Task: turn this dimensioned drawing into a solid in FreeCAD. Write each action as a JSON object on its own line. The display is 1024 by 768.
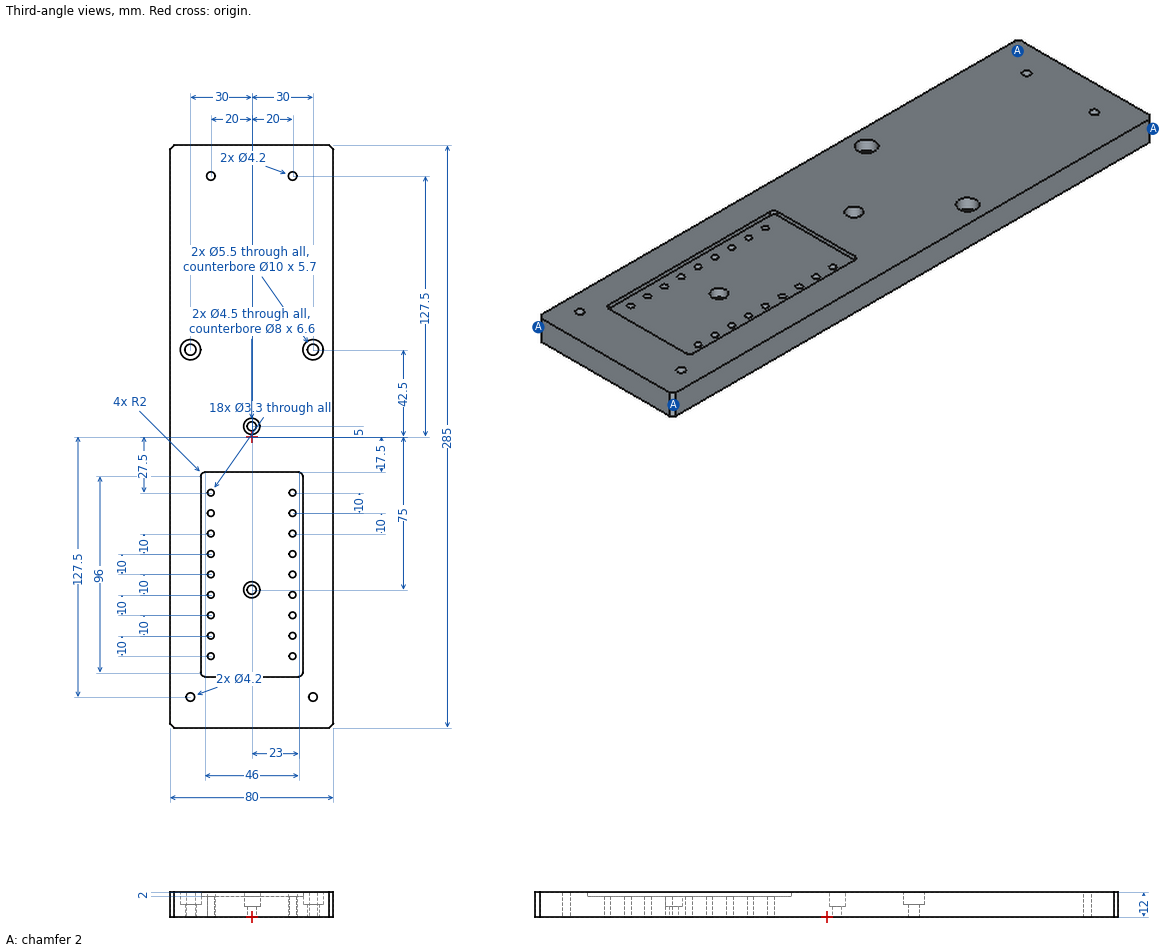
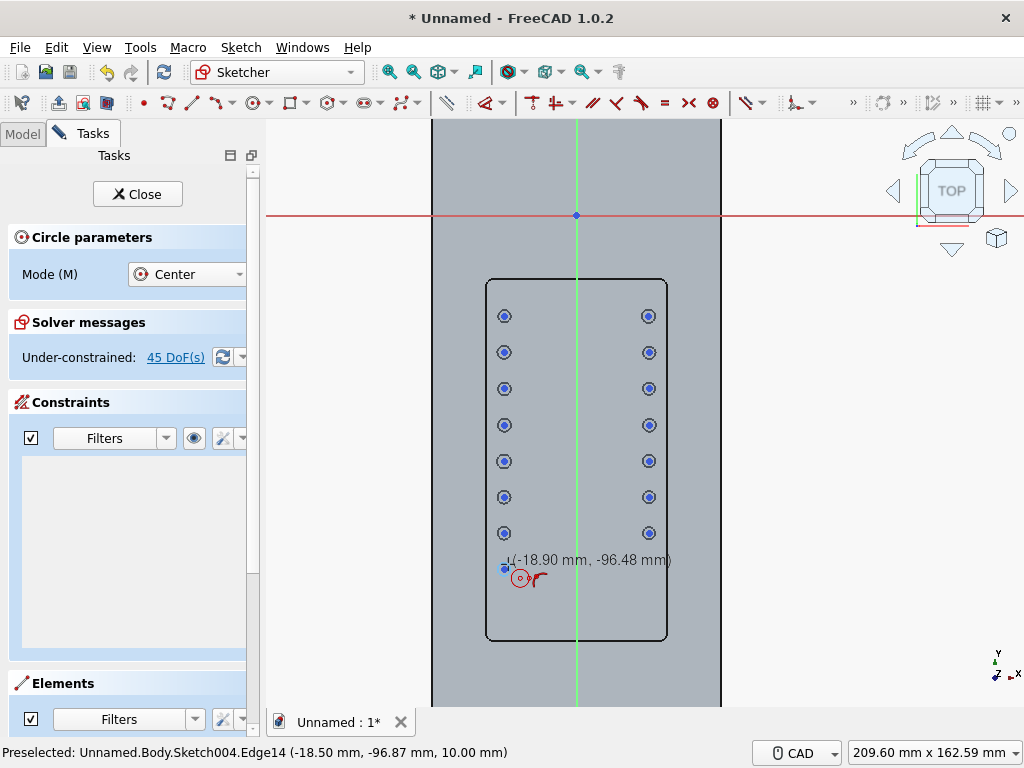
{"action": "scroll", "coordinate": [649, 569], "scroll_direction": "up", "scroll_amount": 7}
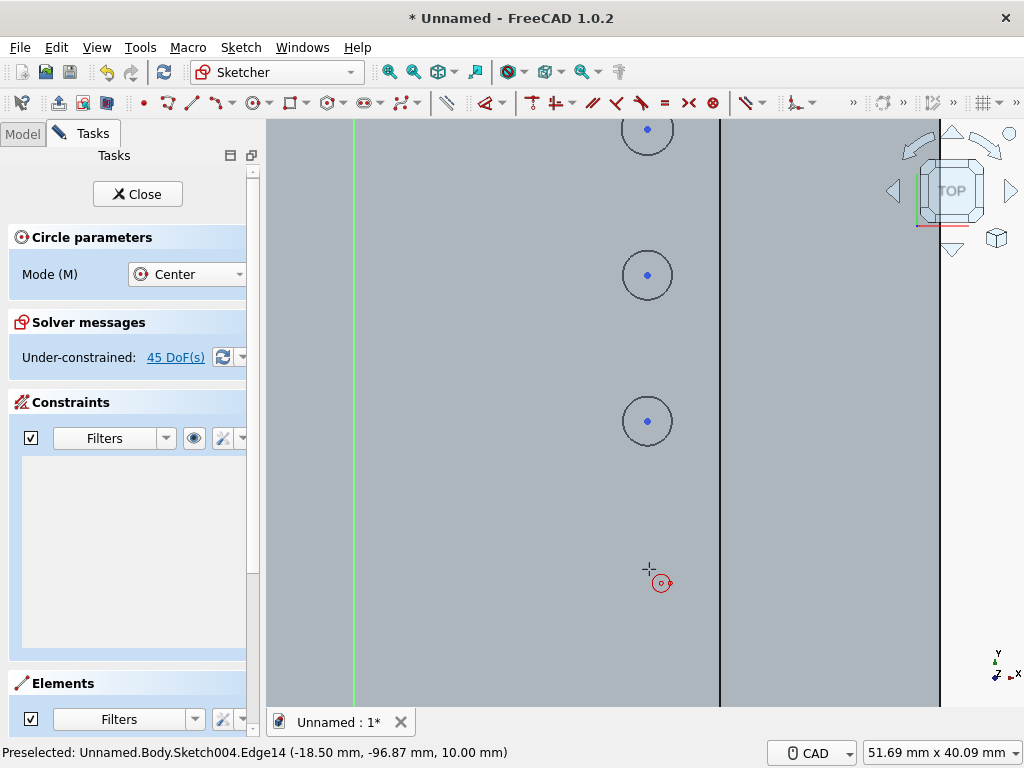
{"action": "scroll", "coordinate": [649, 569], "scroll_direction": "down", "scroll_amount": 7}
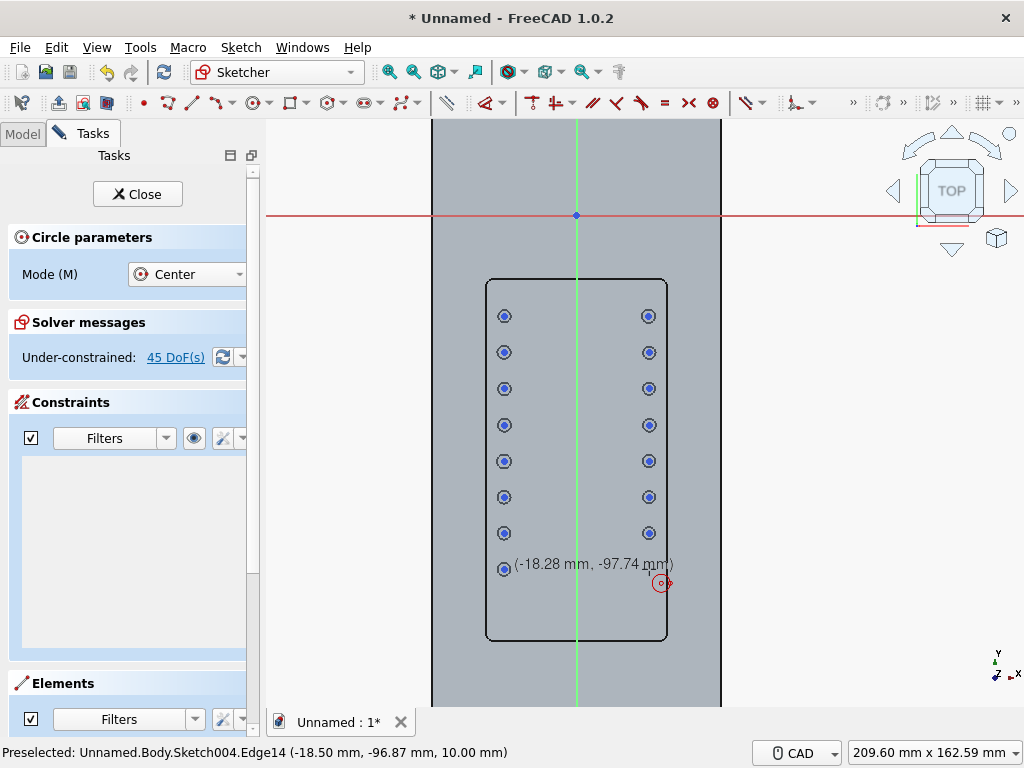
{"action": "left_click", "coordinate": [649, 569]}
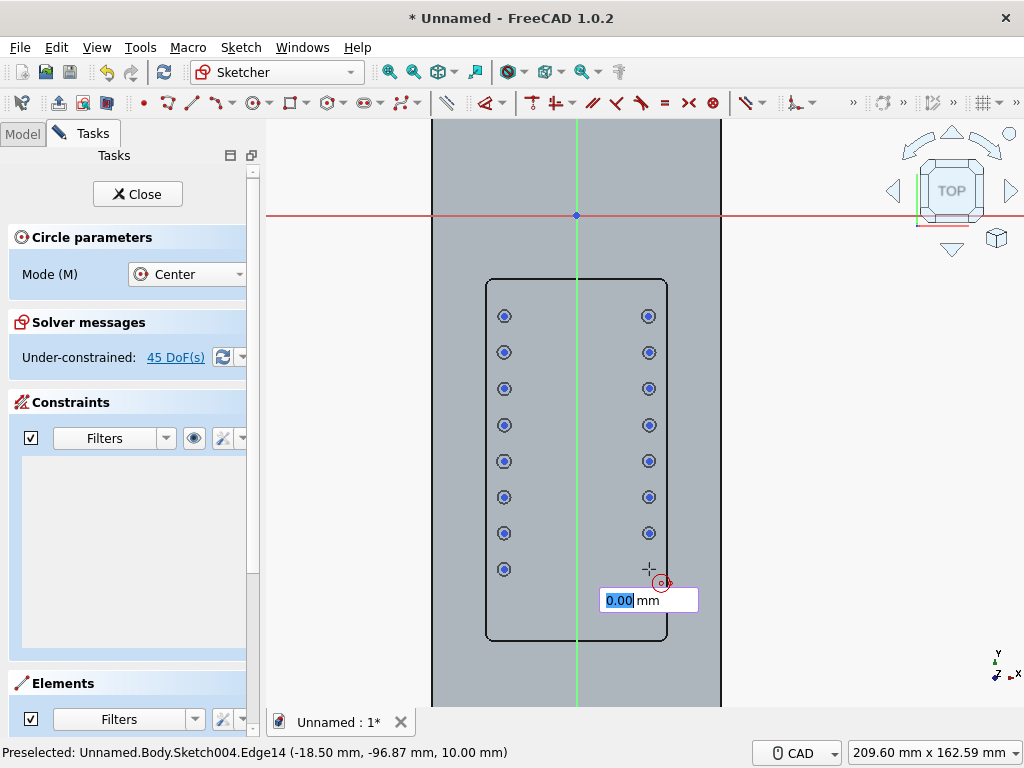
{"action": "scroll", "coordinate": [653, 564], "scroll_direction": "up", "scroll_amount": 5}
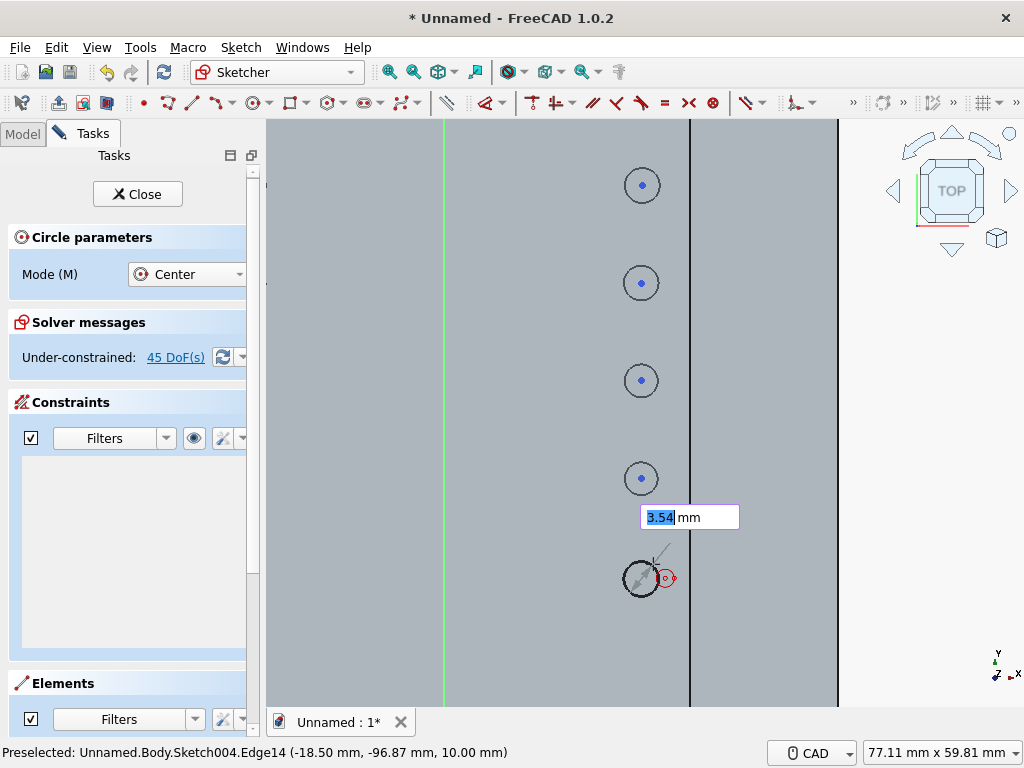
{"action": "left_click", "coordinate": [652, 564]}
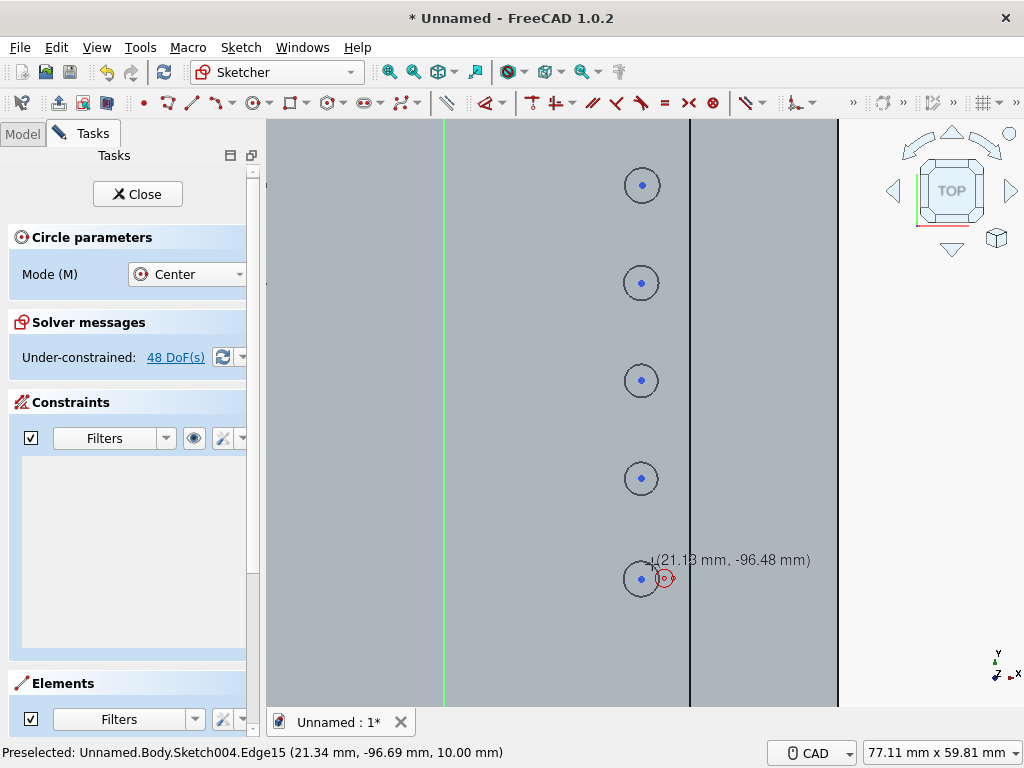
{"action": "scroll", "coordinate": [653, 564], "scroll_direction": "down", "scroll_amount": 5}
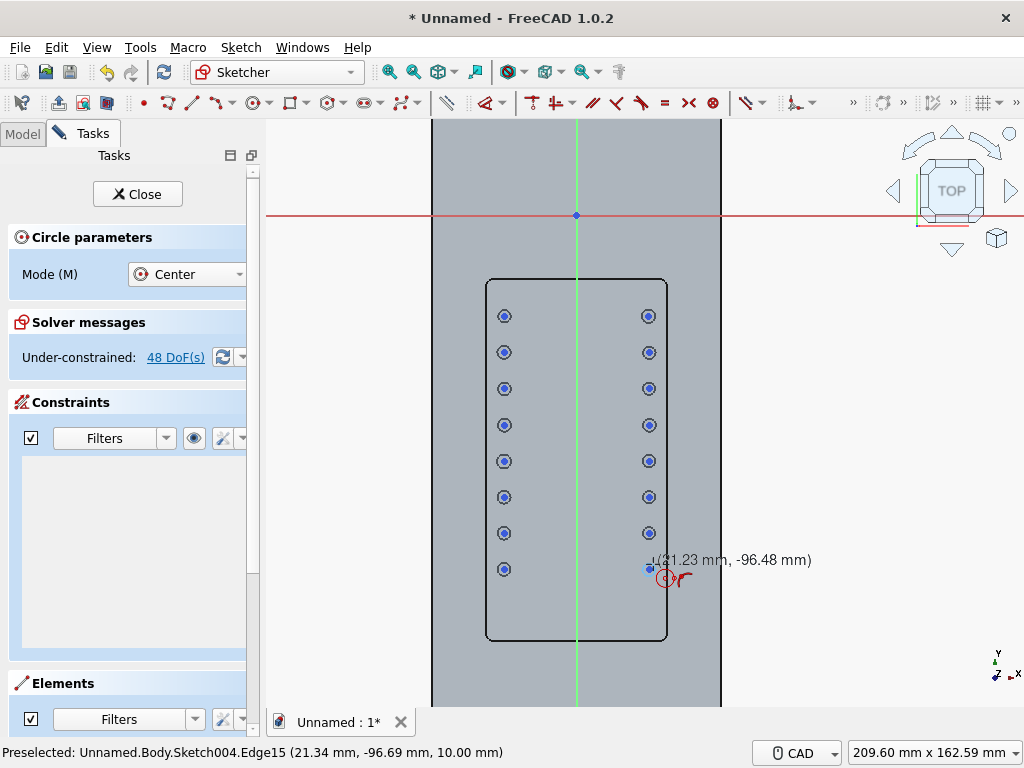
{"action": "scroll", "coordinate": [504, 605], "scroll_direction": "up", "scroll_amount": 7}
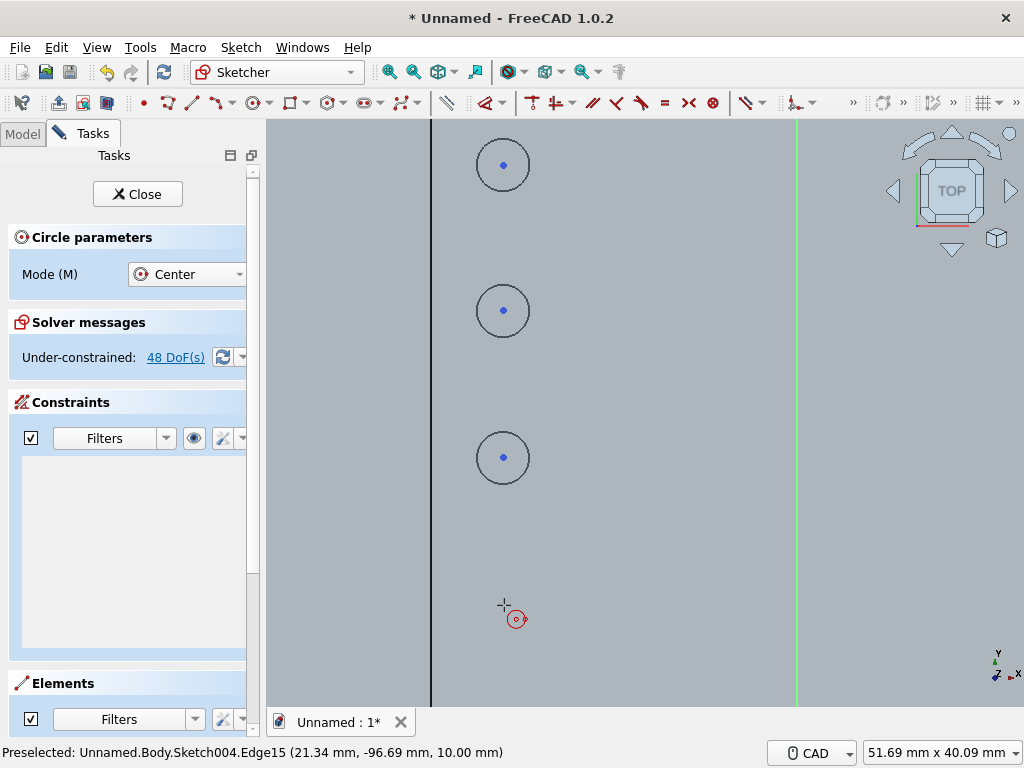
{"action": "scroll", "coordinate": [504, 605], "scroll_direction": "down", "scroll_amount": 7}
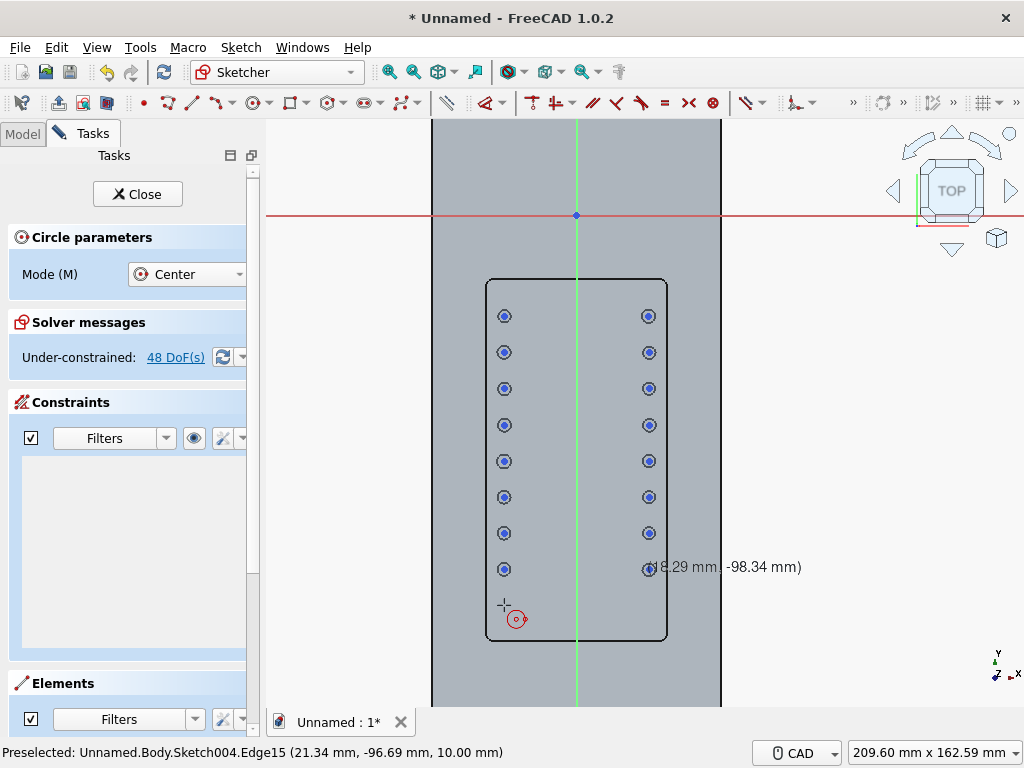
{"action": "left_click", "coordinate": [504, 605]}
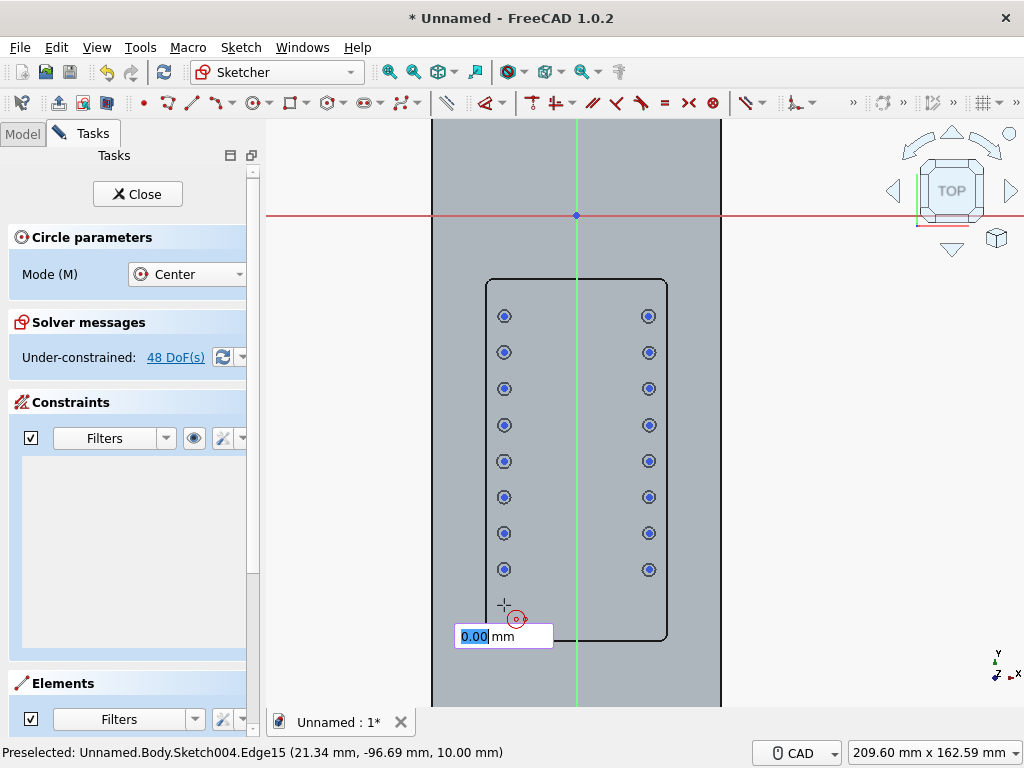
{"action": "scroll", "coordinate": [508, 600], "scroll_direction": "up", "scroll_amount": 5}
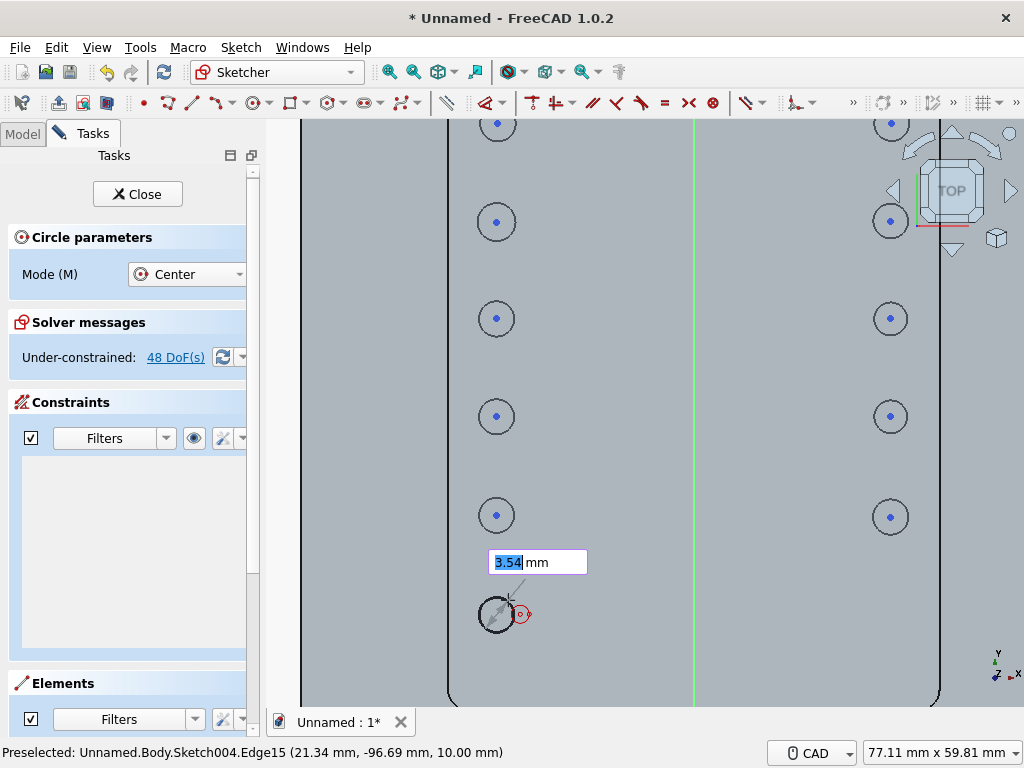
{"action": "left_click", "coordinate": [509, 600]}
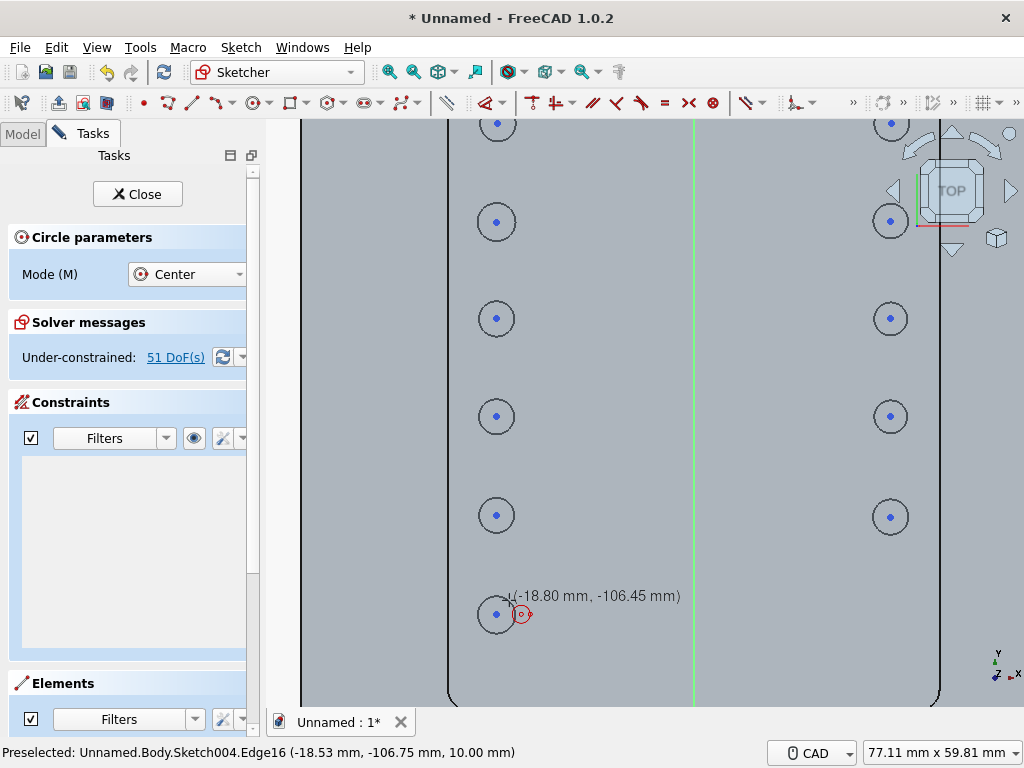
{"action": "scroll", "coordinate": [508, 600], "scroll_direction": "down", "scroll_amount": 5}